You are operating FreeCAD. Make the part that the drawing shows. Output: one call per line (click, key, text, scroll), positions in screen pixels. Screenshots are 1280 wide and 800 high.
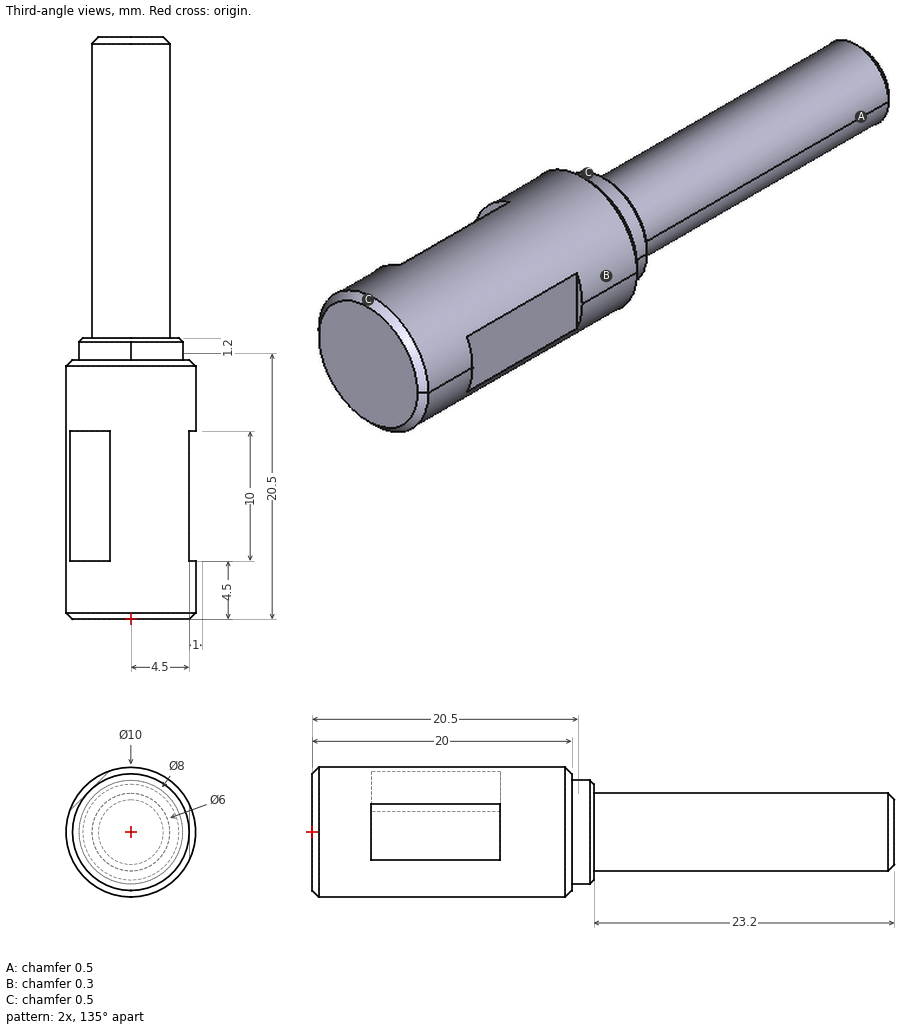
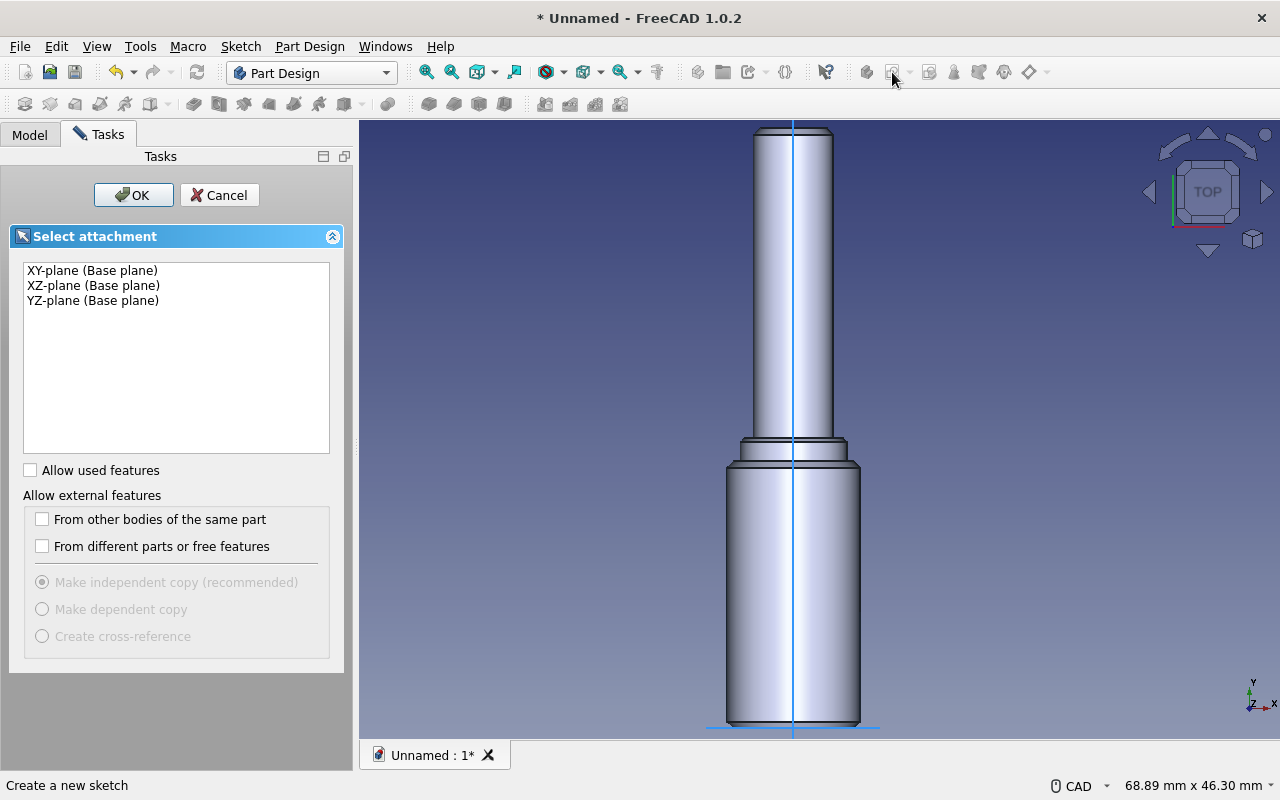
click(84, 270)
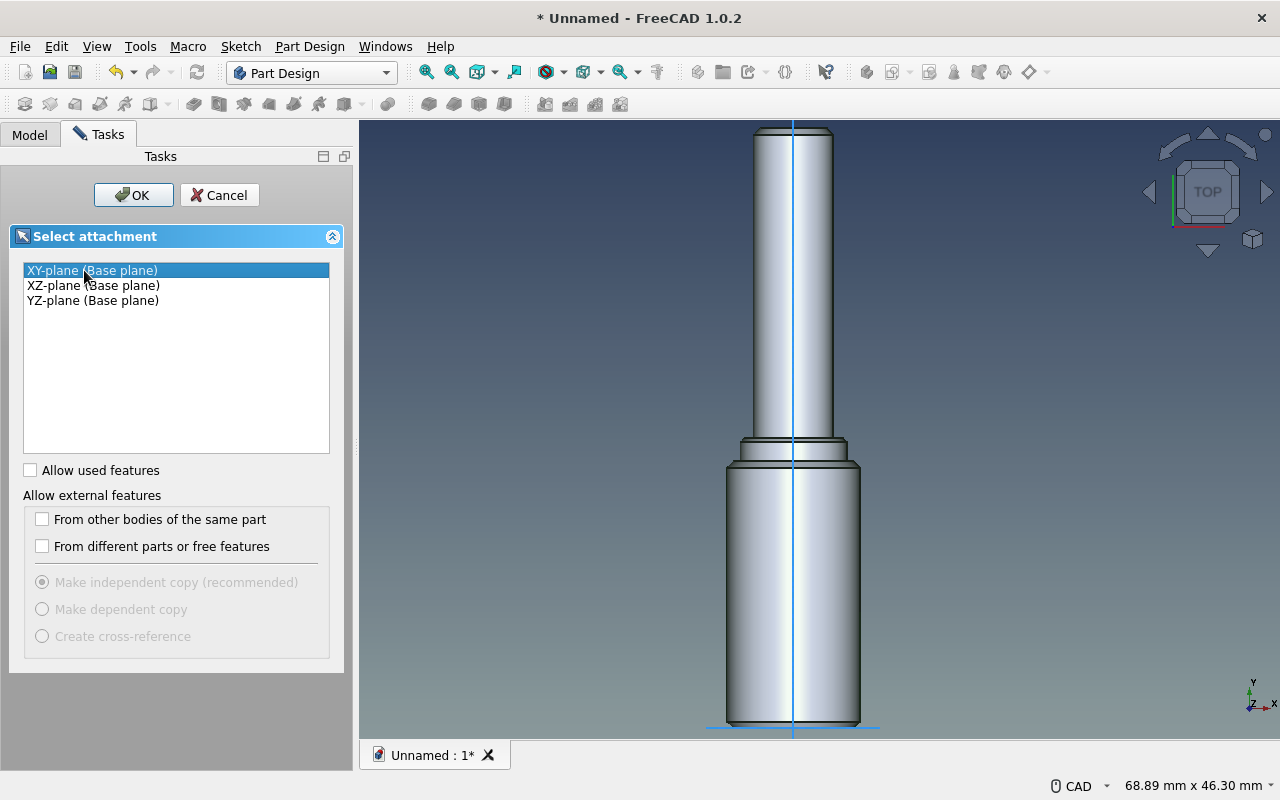
click(134, 195)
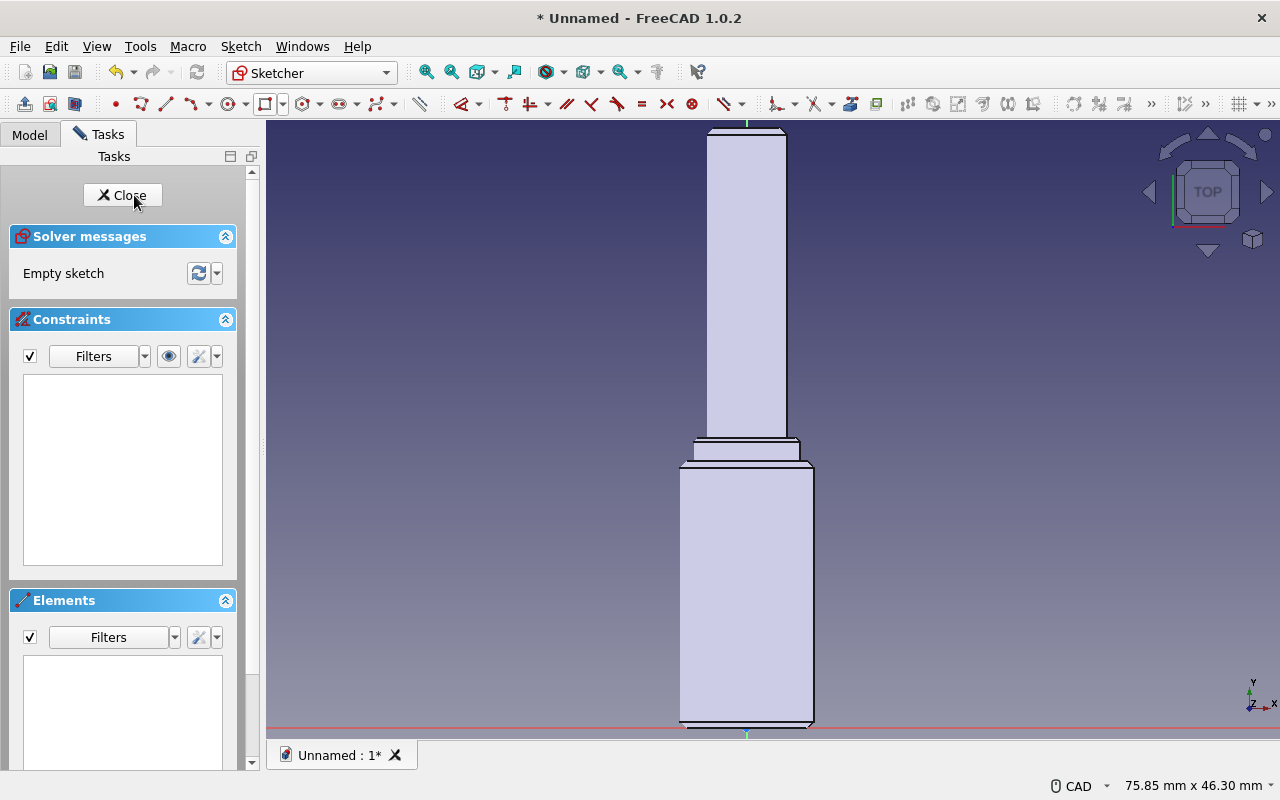
click(75, 104)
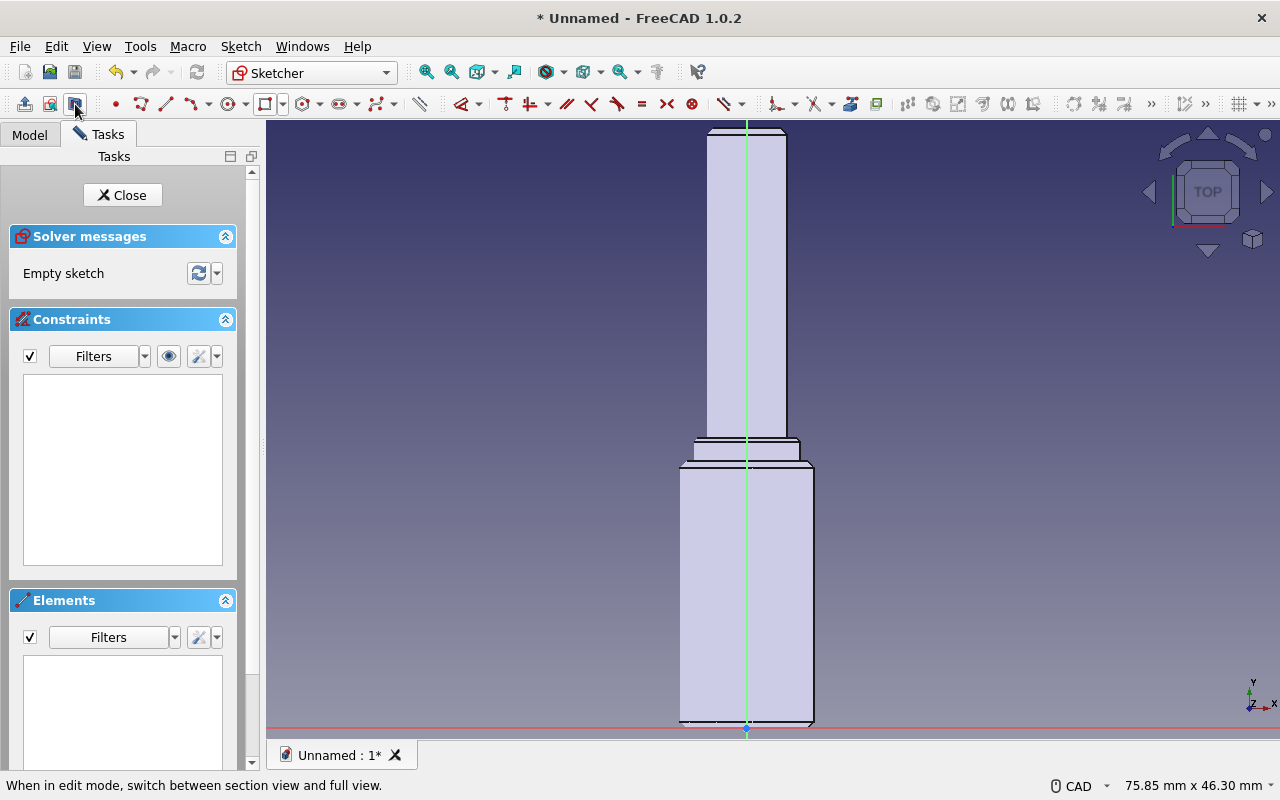
scroll(704, 430, down, 5)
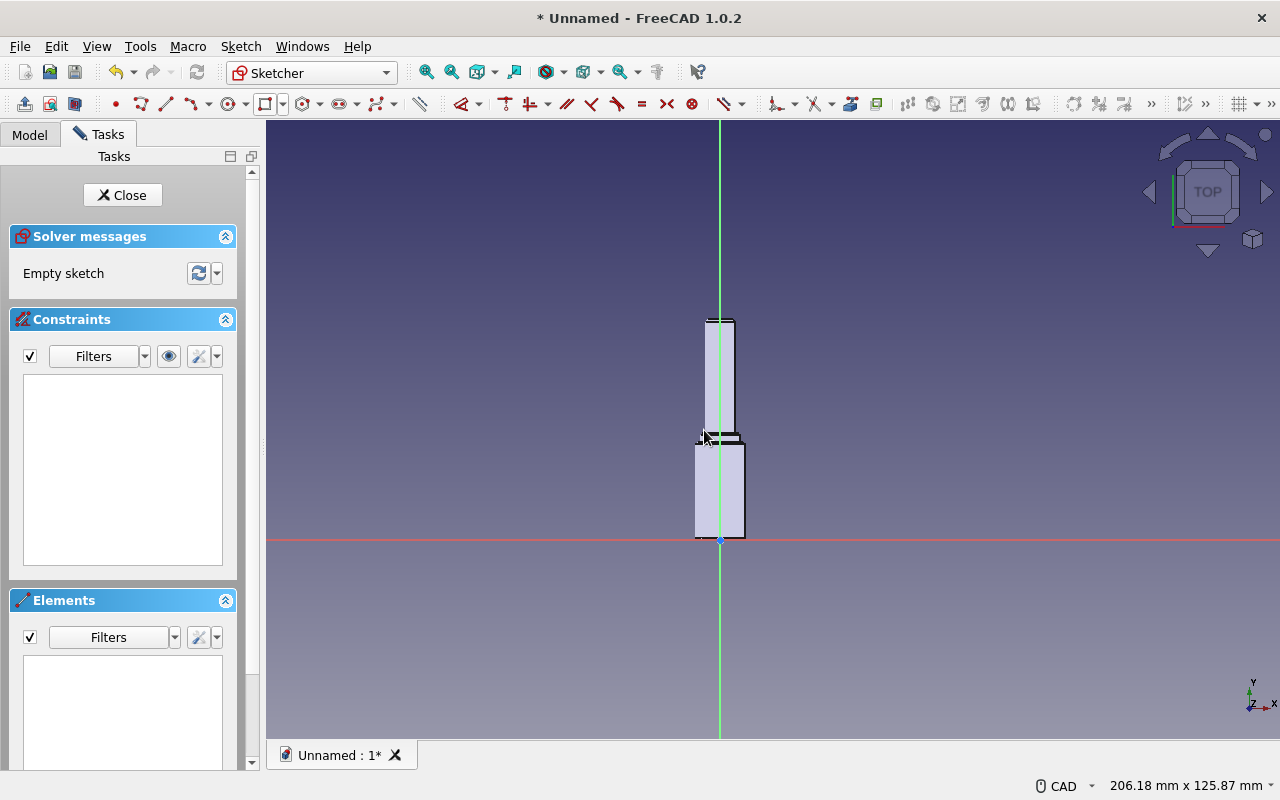
scroll(739, 519, up, 9)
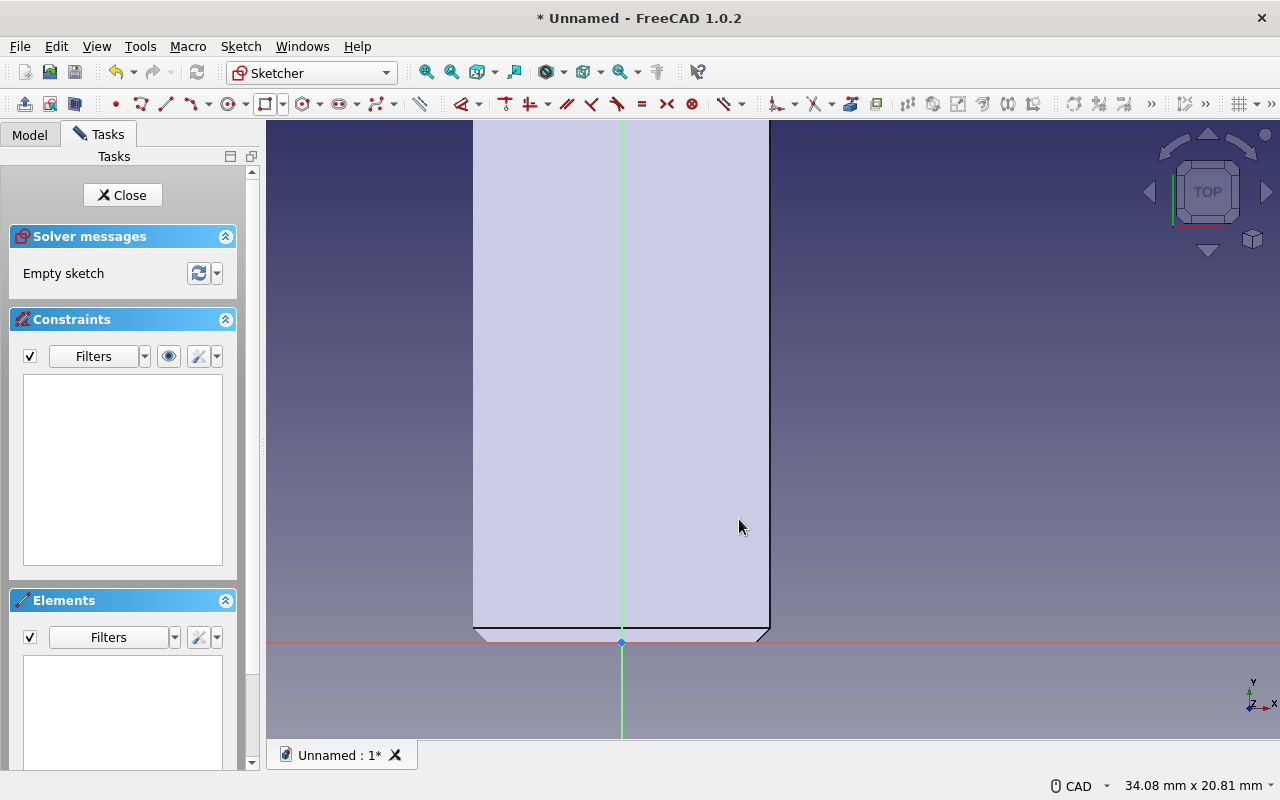
click(264, 104)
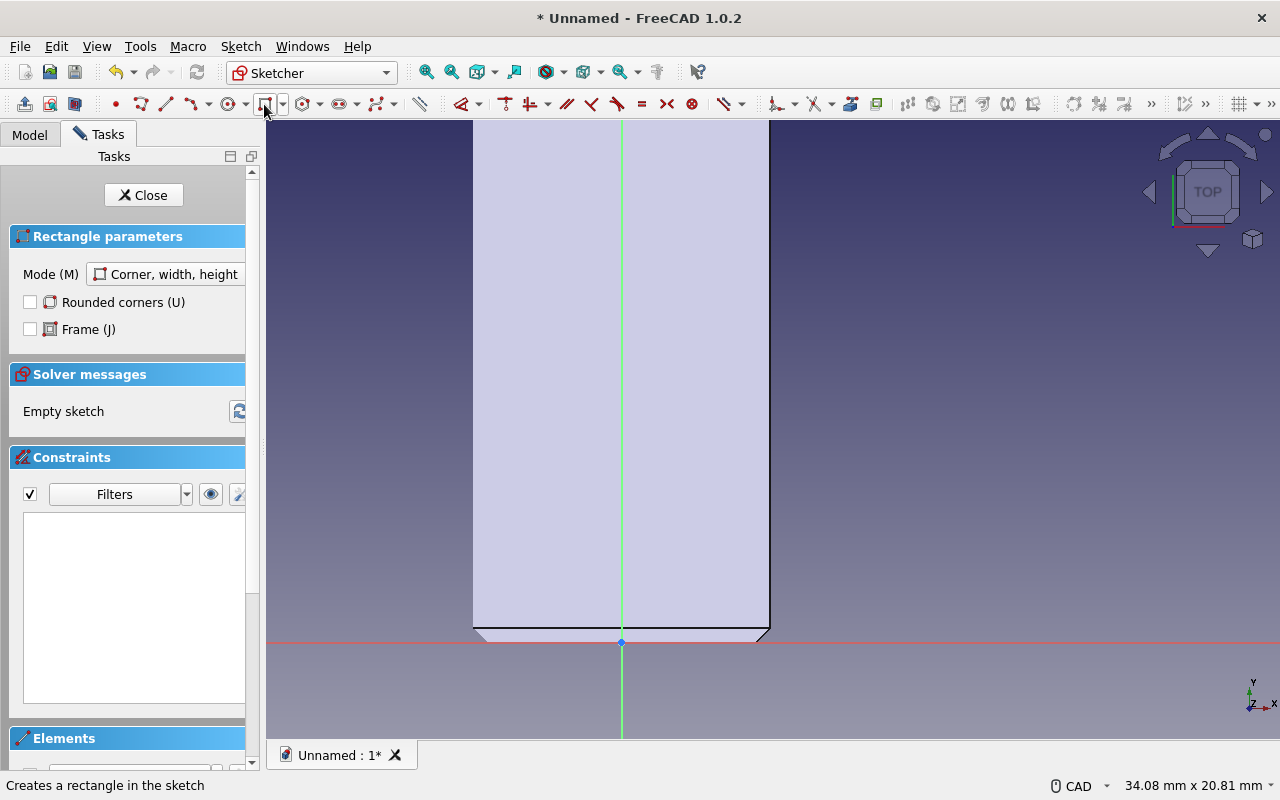
click(756, 211)
move(785, 509)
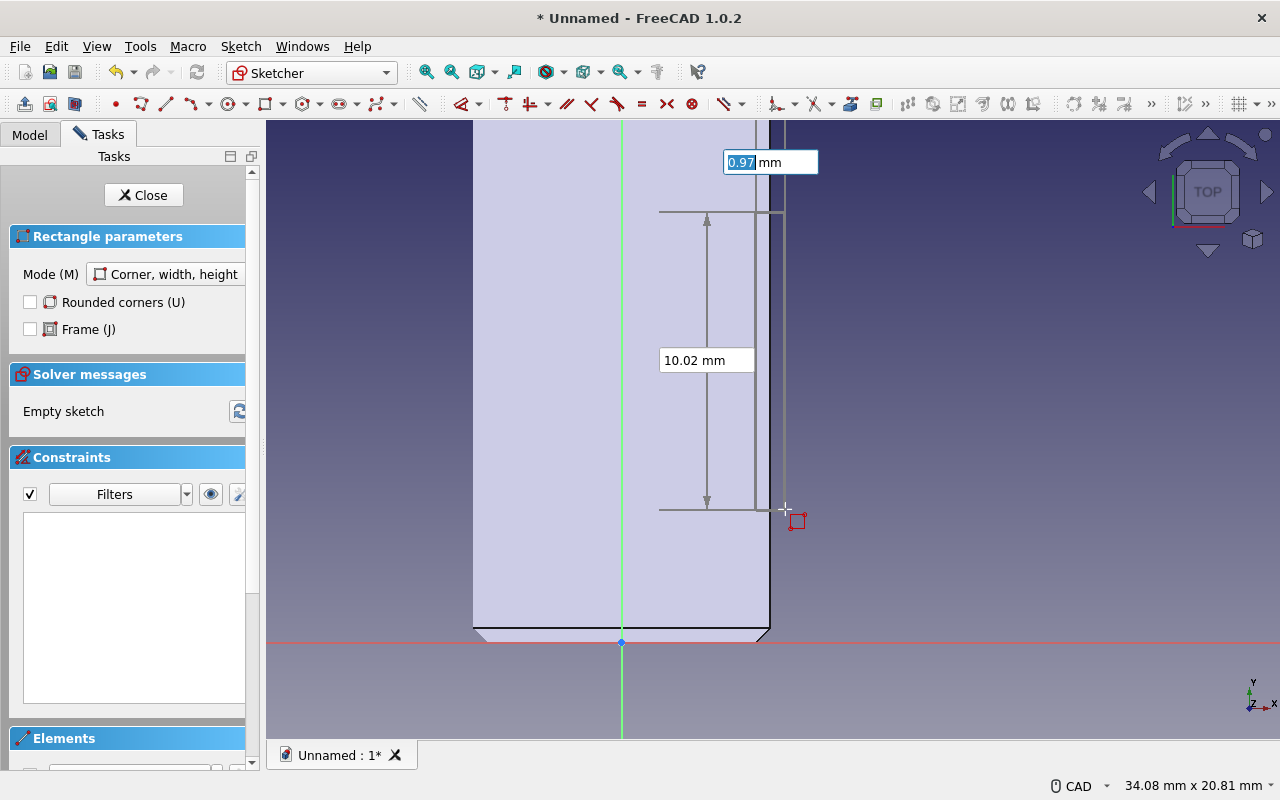
text(1)
key(Tab)
text(10)
key(Return)
key(Escape)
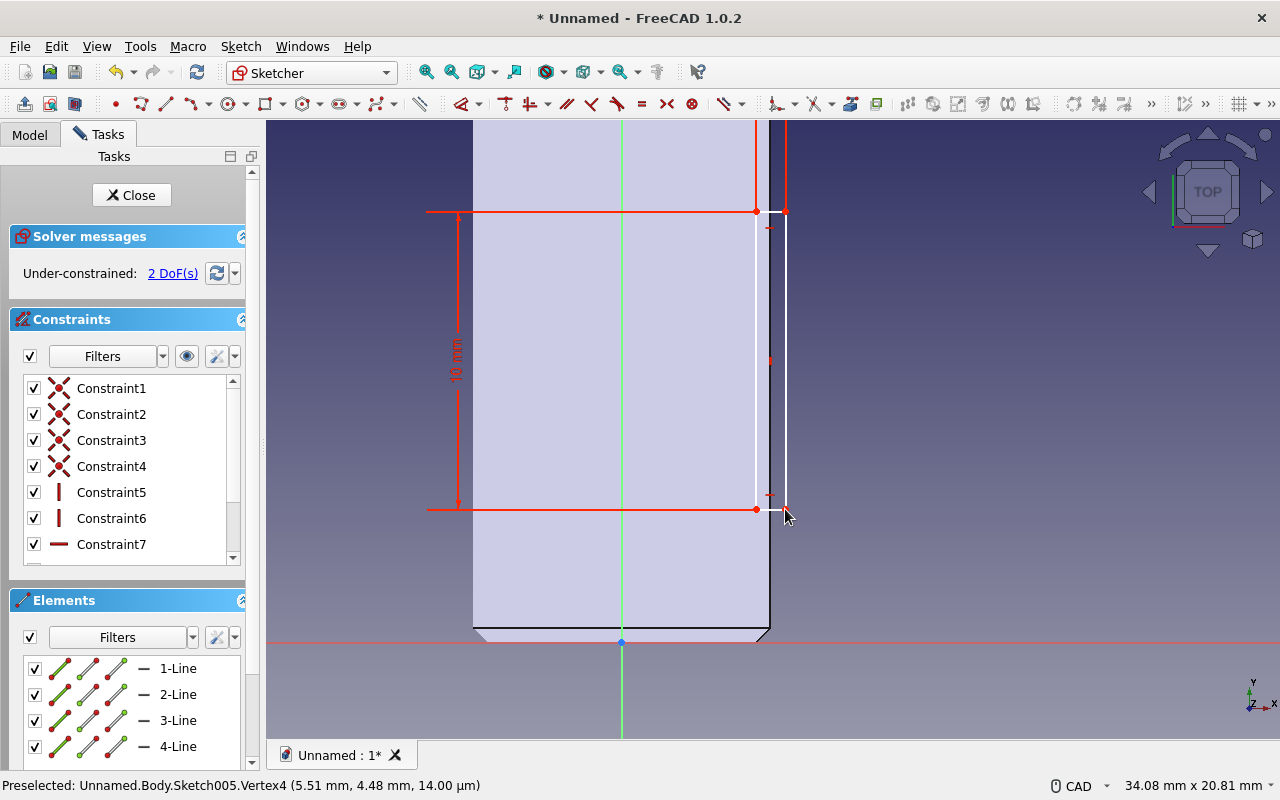
click(460, 104)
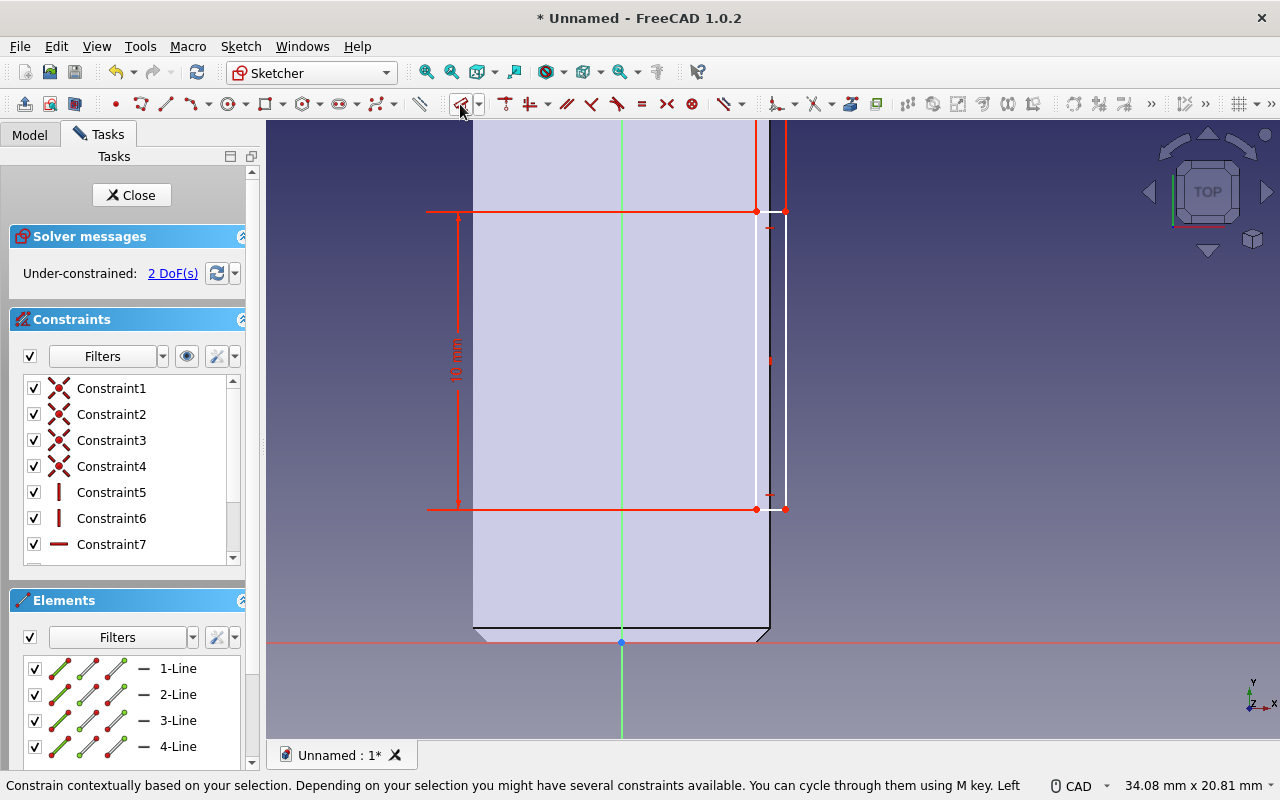
click(756, 212)
click(689, 677)